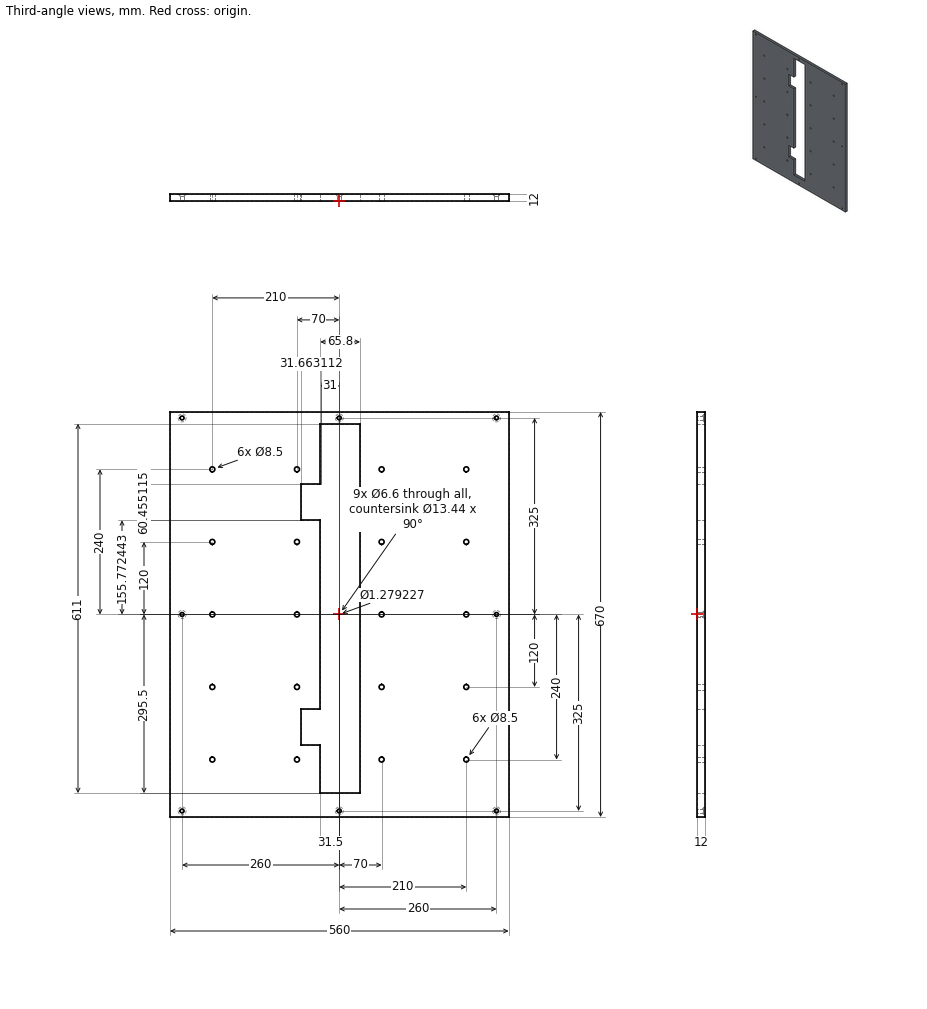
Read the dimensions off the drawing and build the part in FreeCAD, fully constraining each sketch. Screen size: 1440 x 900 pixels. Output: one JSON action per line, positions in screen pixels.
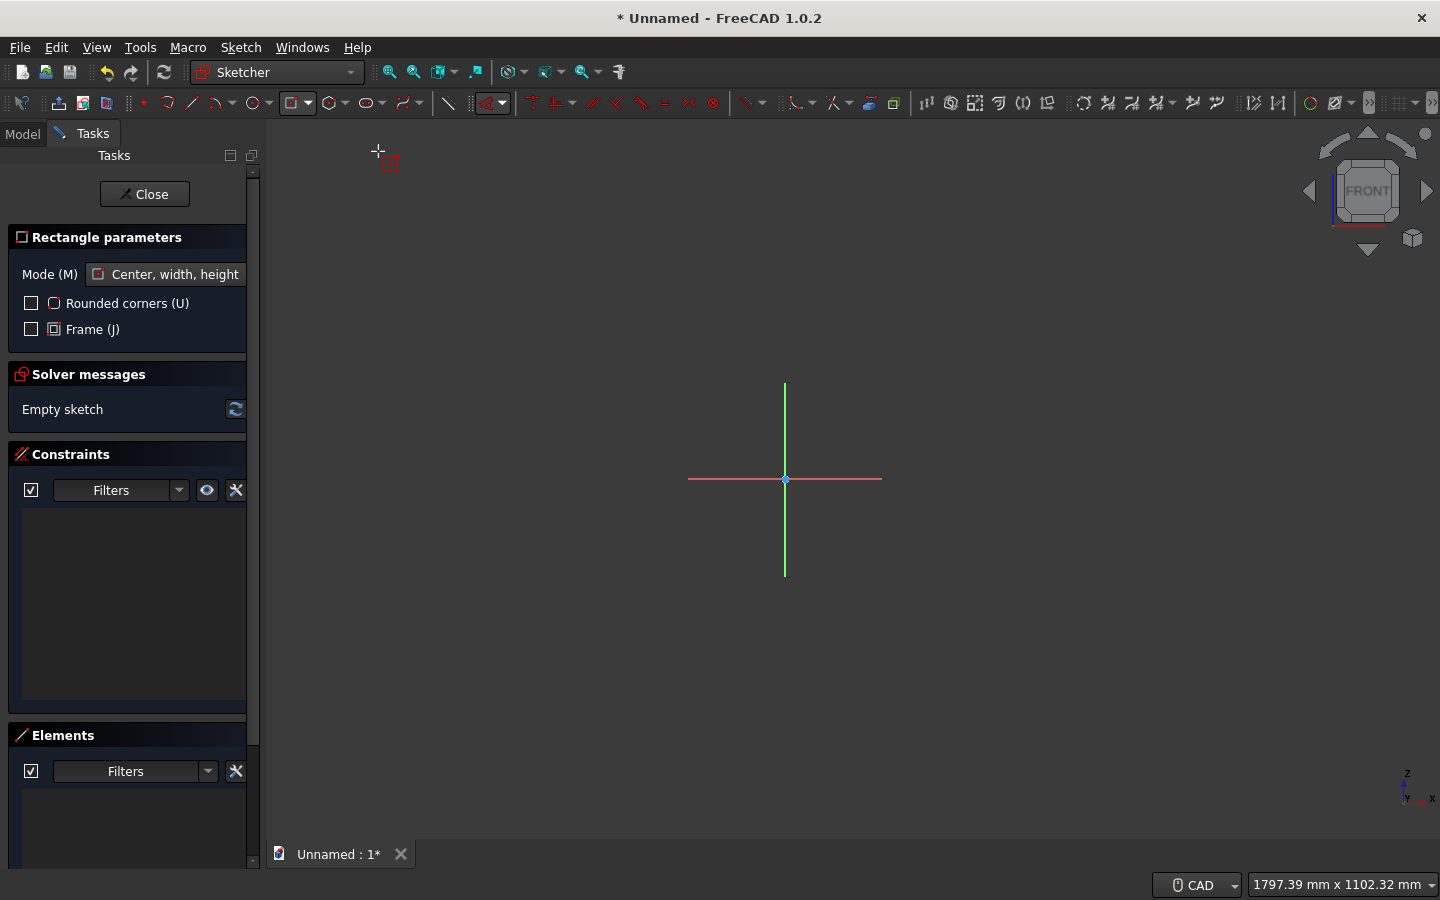
{"action": "left_click", "coordinate": [785, 479]}
{"action": "left_click", "coordinate": [968, 261]}
{"action": "key", "text": "Escape"}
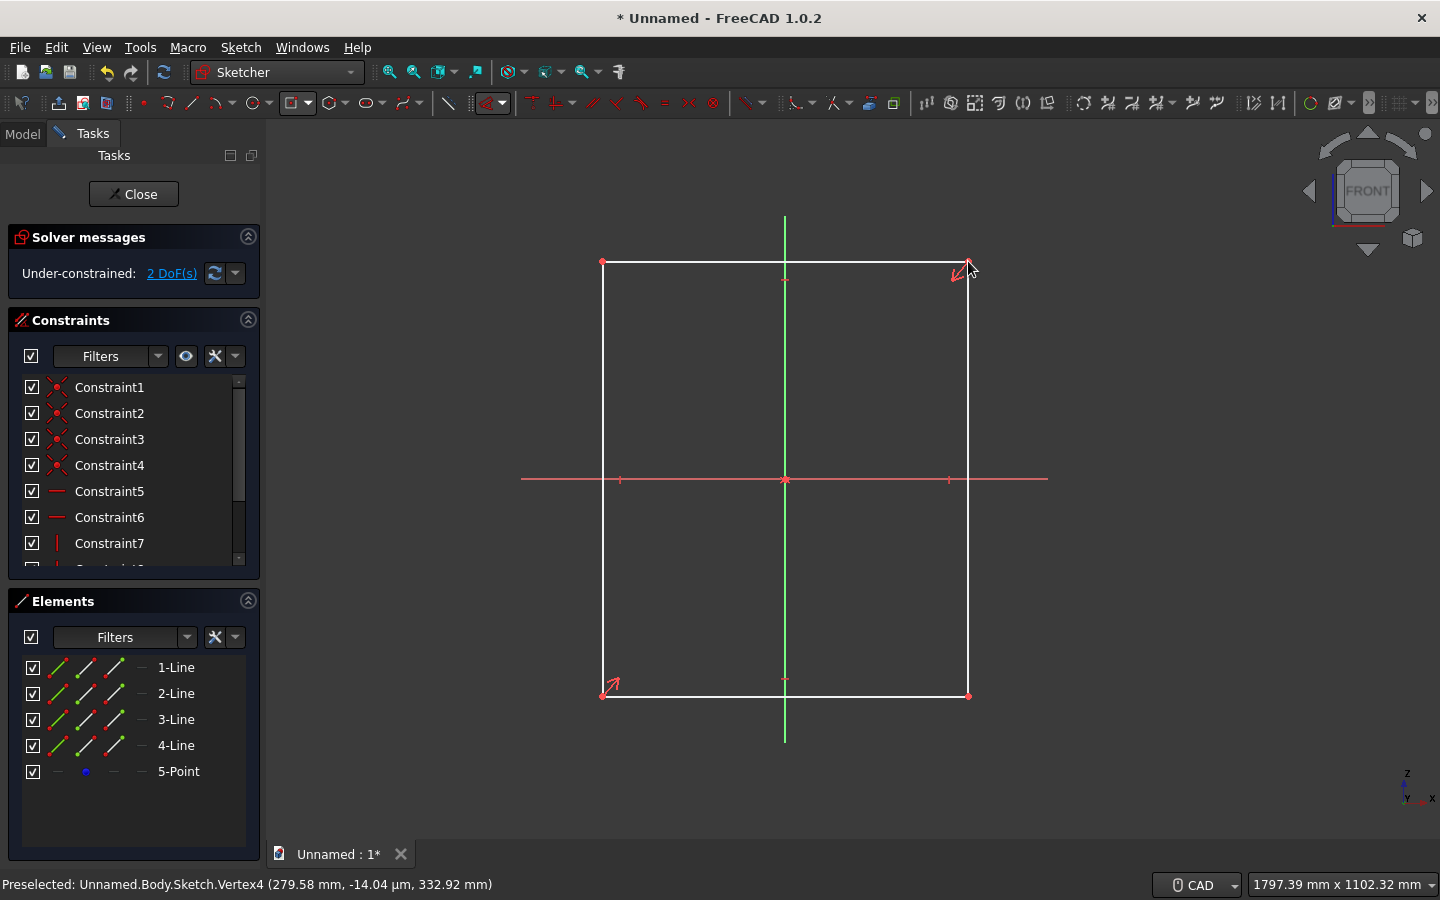
{"action": "left_click", "coordinate": [486, 104]}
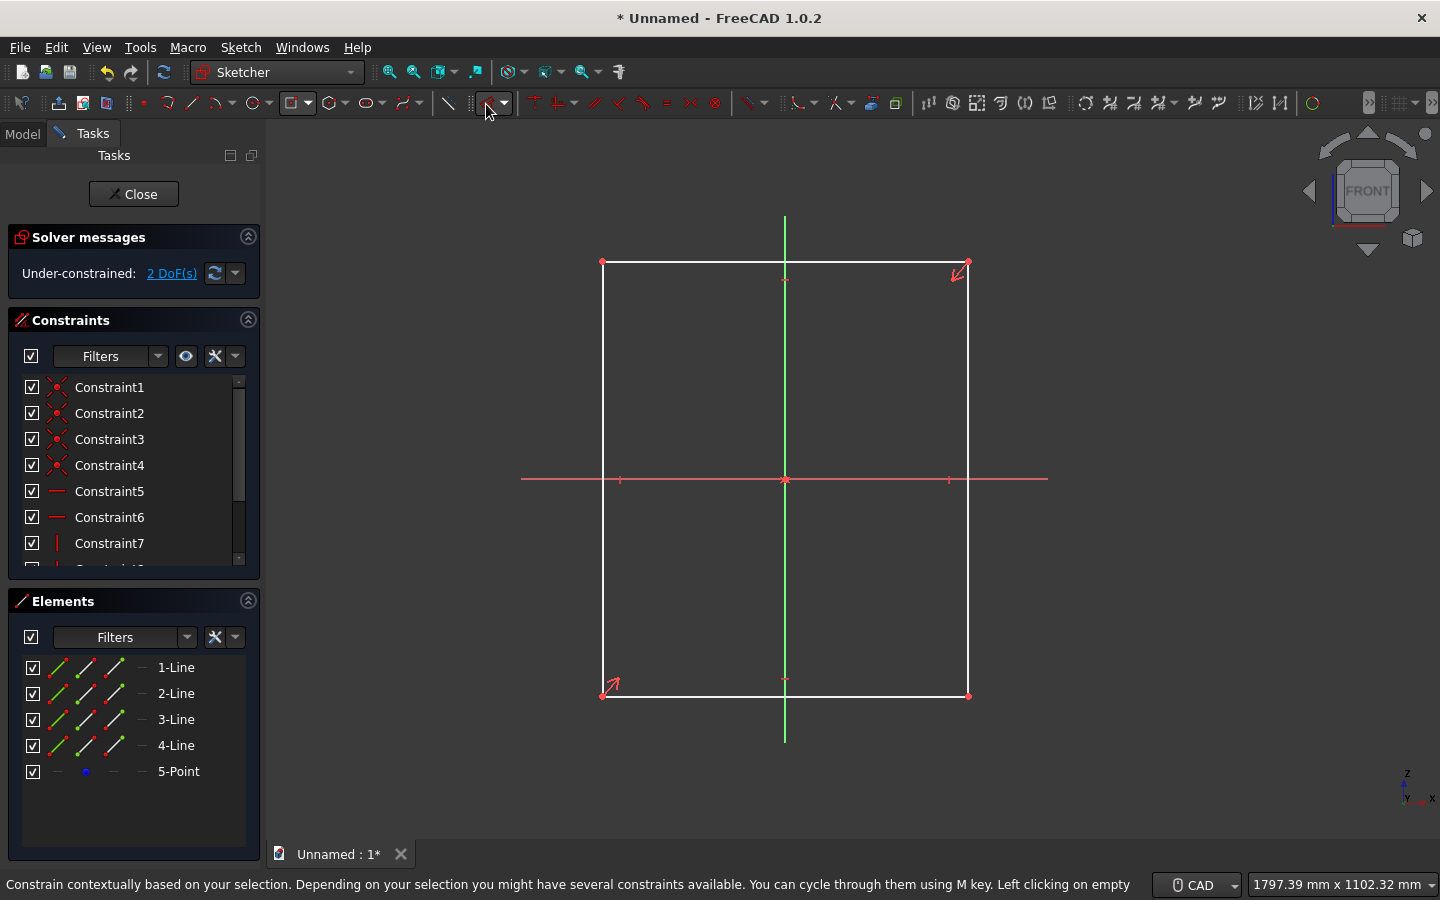
{"action": "left_click", "coordinate": [712, 697]}
{"action": "left_click", "coordinate": [701, 731]}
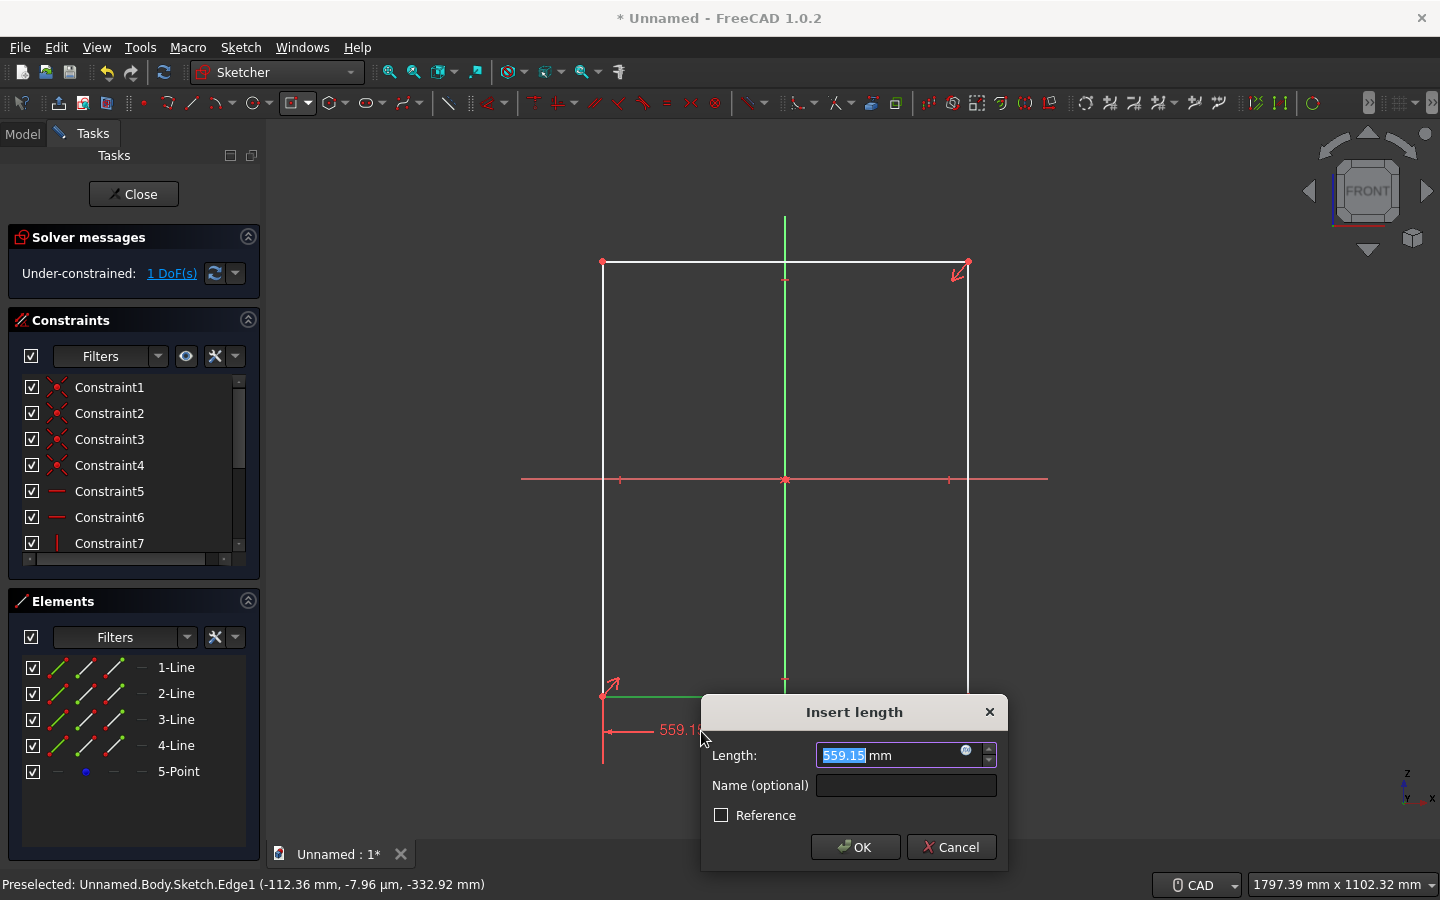
{"action": "type", "text": "560"}
{"action": "key", "text": "Return"}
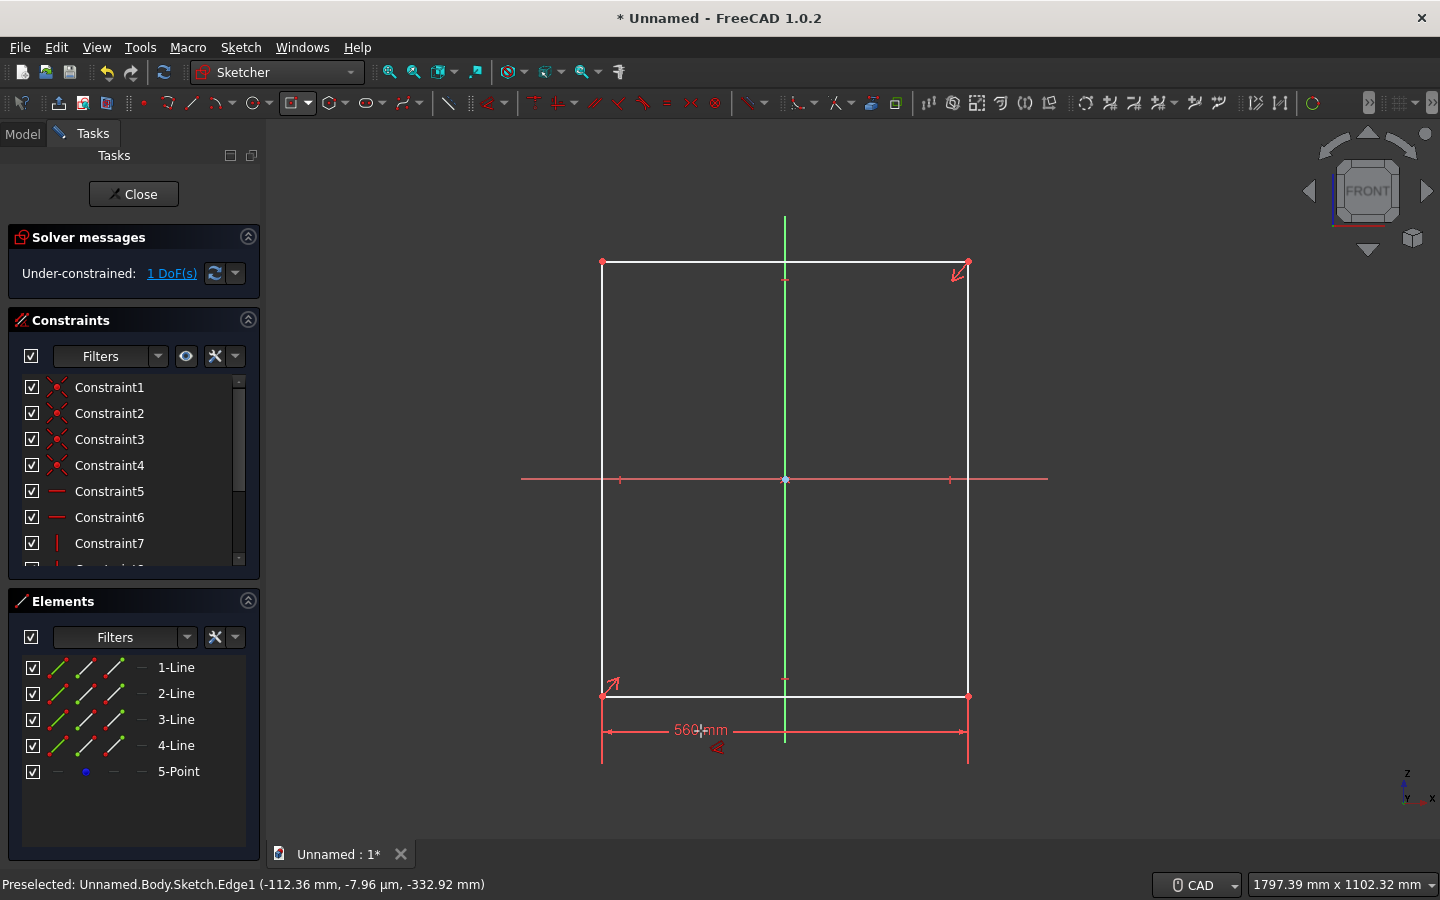
{"action": "left_click", "coordinate": [968, 566]}
{"action": "left_click", "coordinate": [1002, 379]}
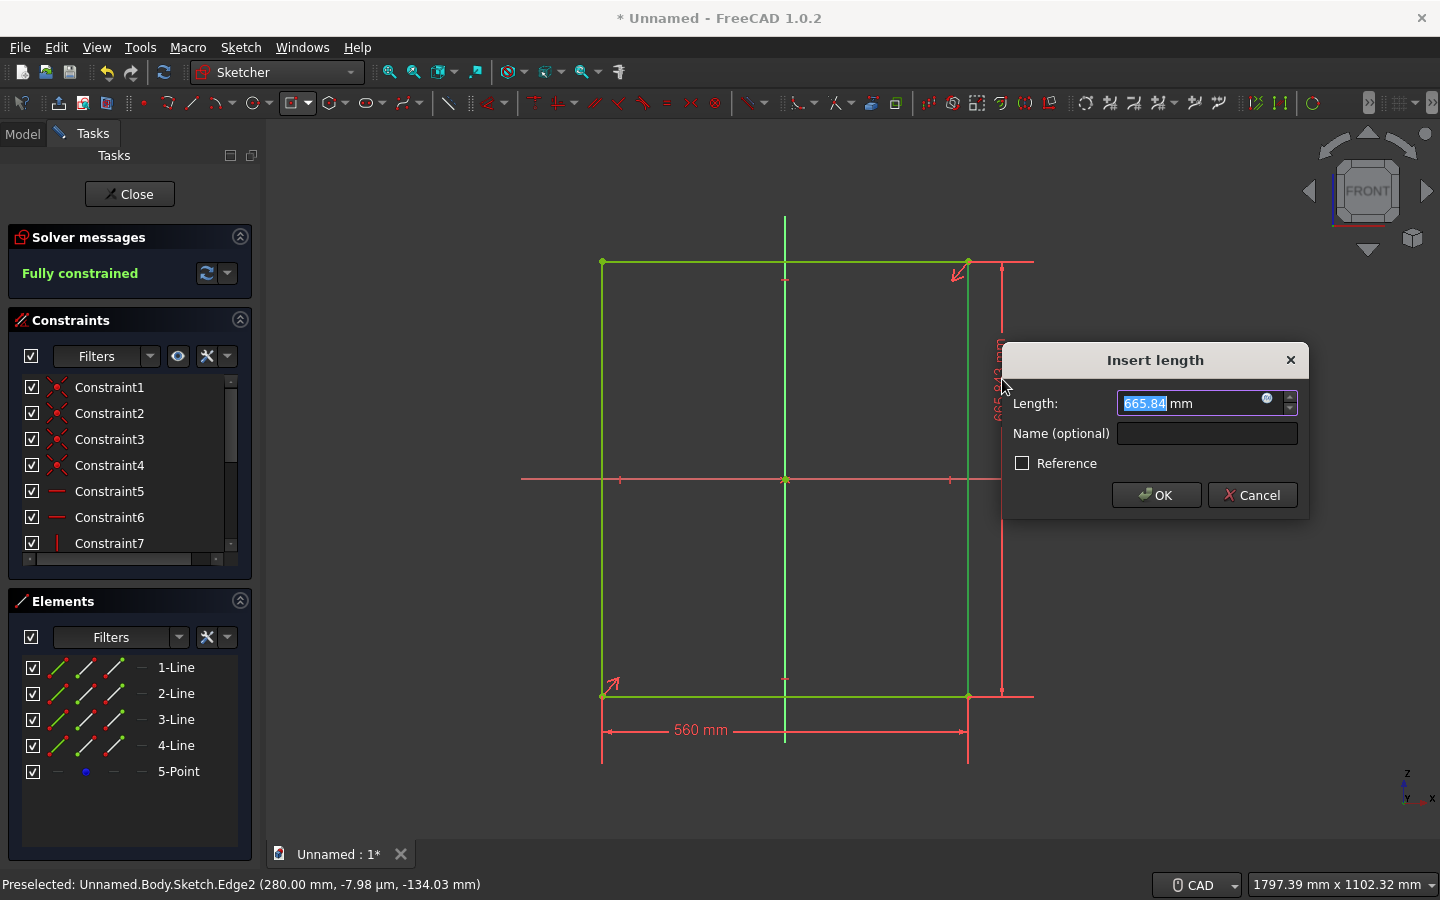
{"action": "type", "text": "670"}
{"action": "key", "text": "Return"}
{"action": "key", "text": "Escape"}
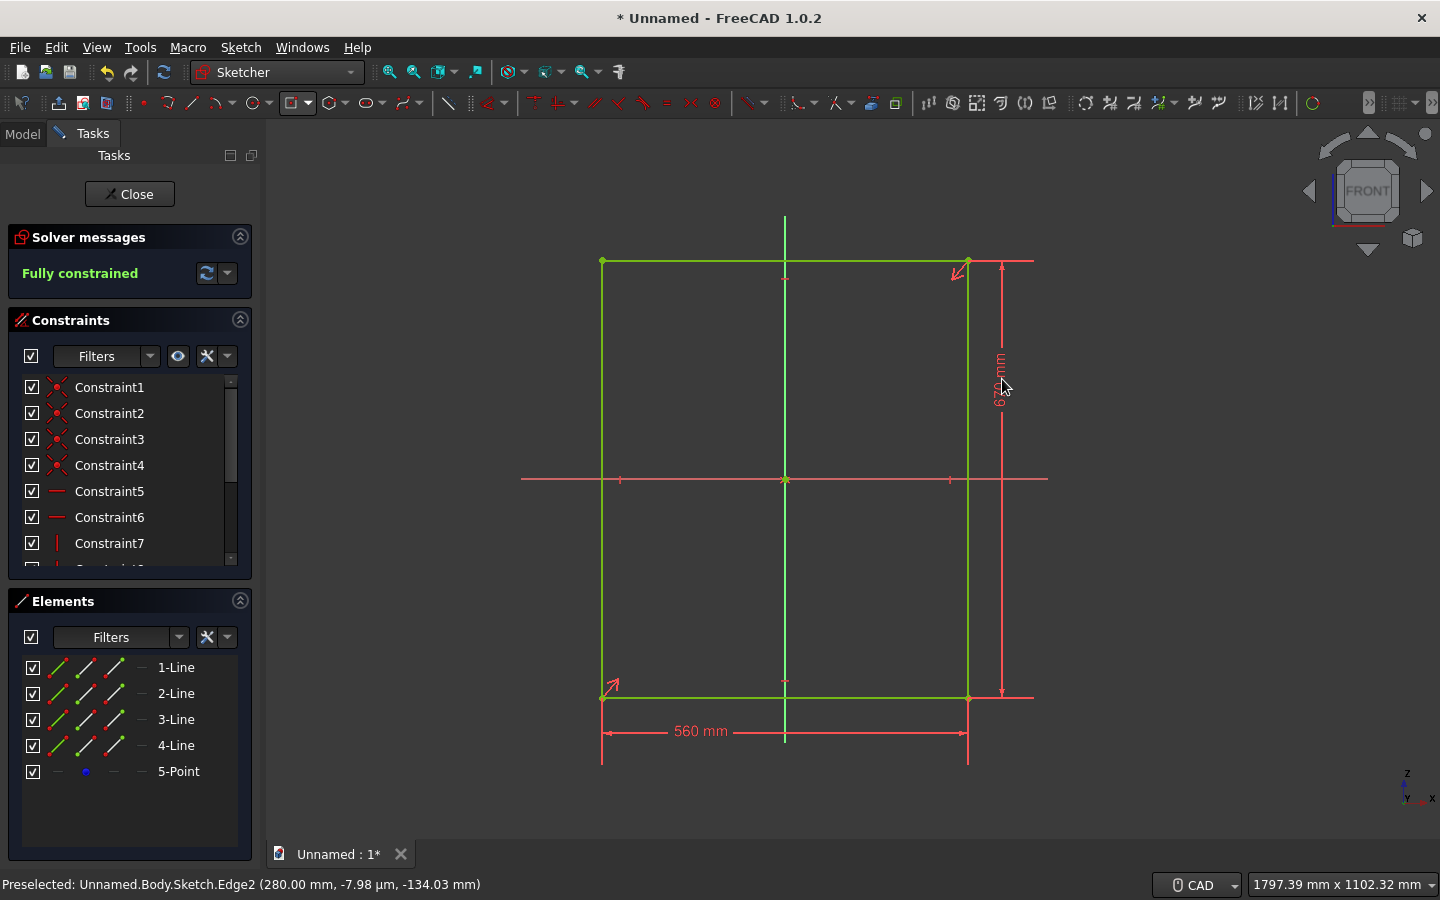
{"action": "left_click", "coordinate": [130, 194]}